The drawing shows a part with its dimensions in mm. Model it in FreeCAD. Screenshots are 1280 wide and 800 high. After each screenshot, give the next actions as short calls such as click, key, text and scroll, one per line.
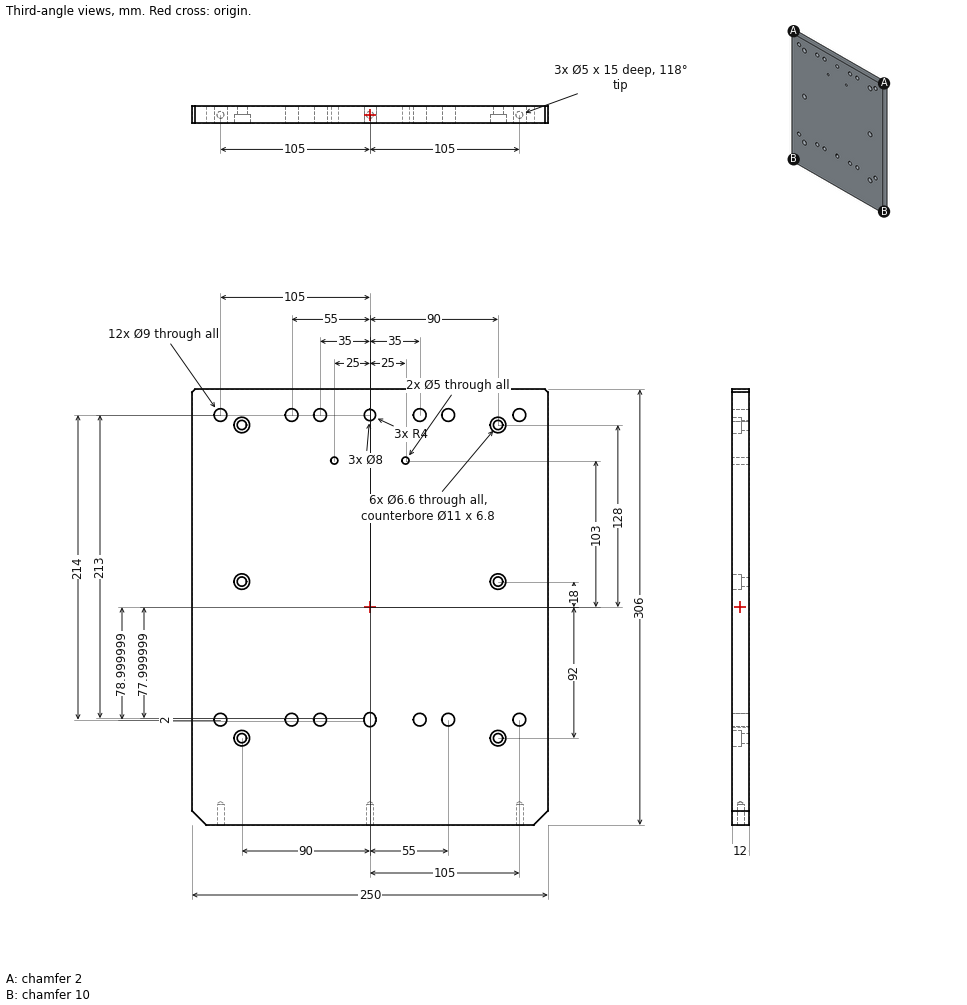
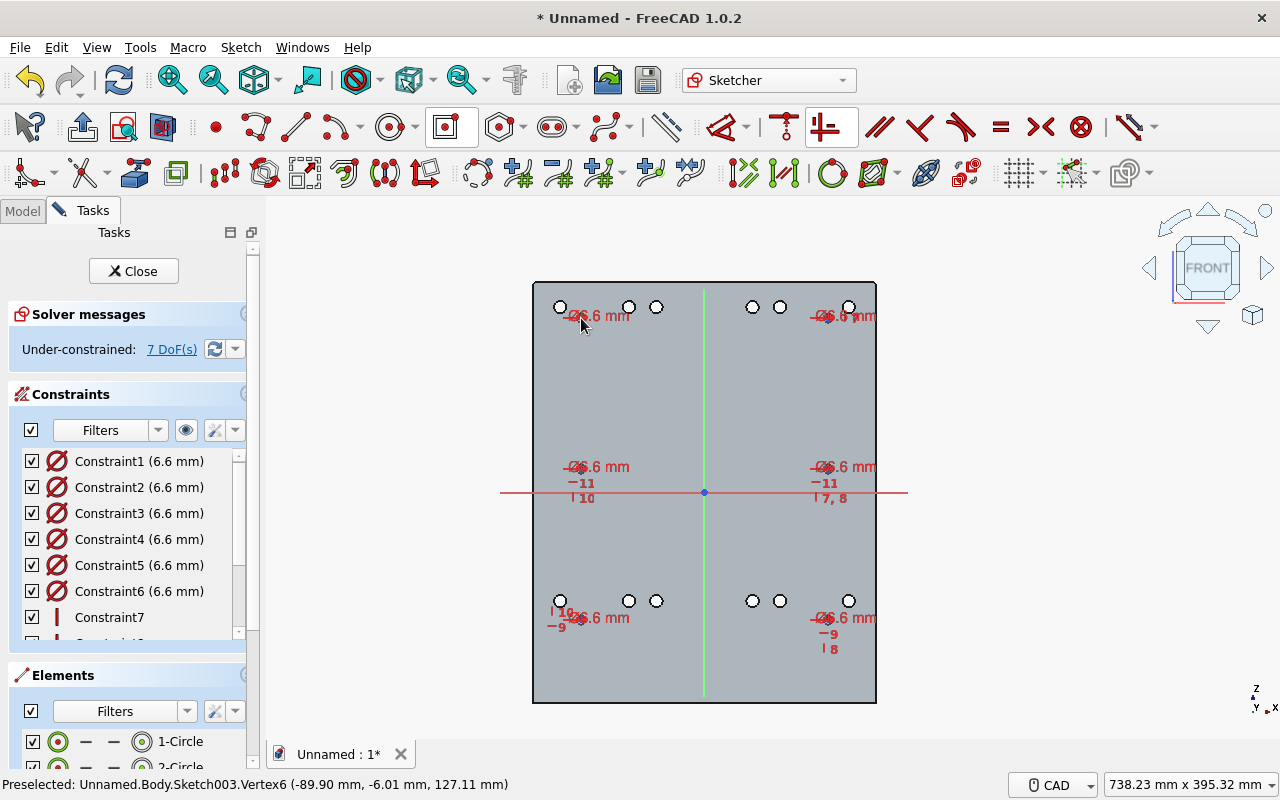
click(852, 128)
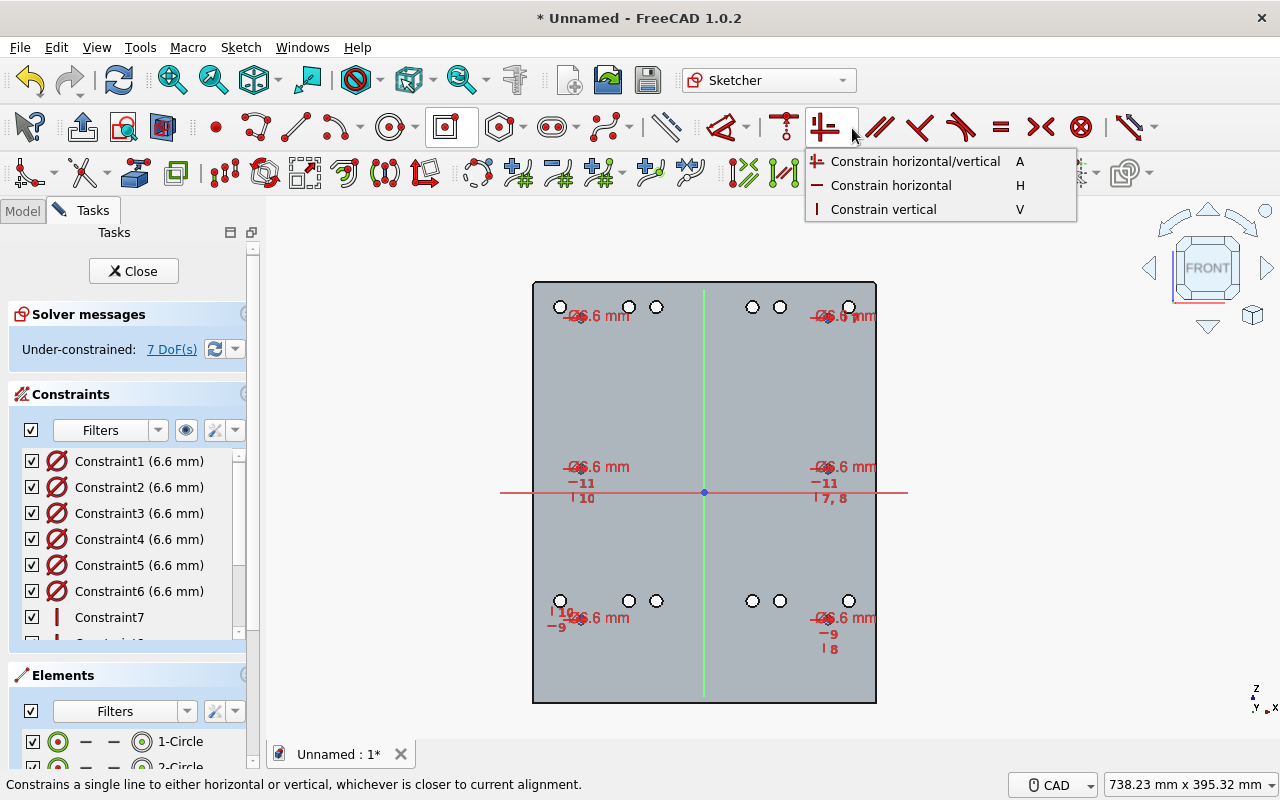
click(941, 209)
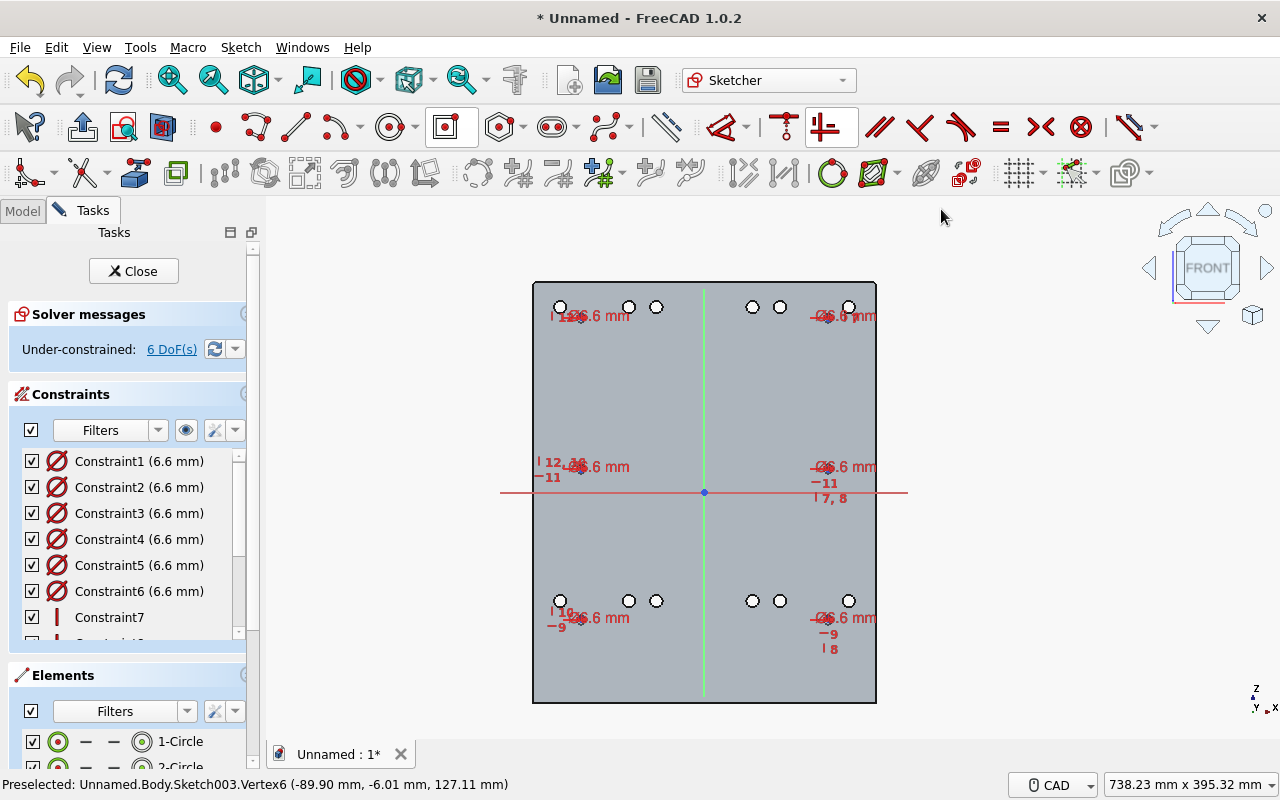
click(828, 318)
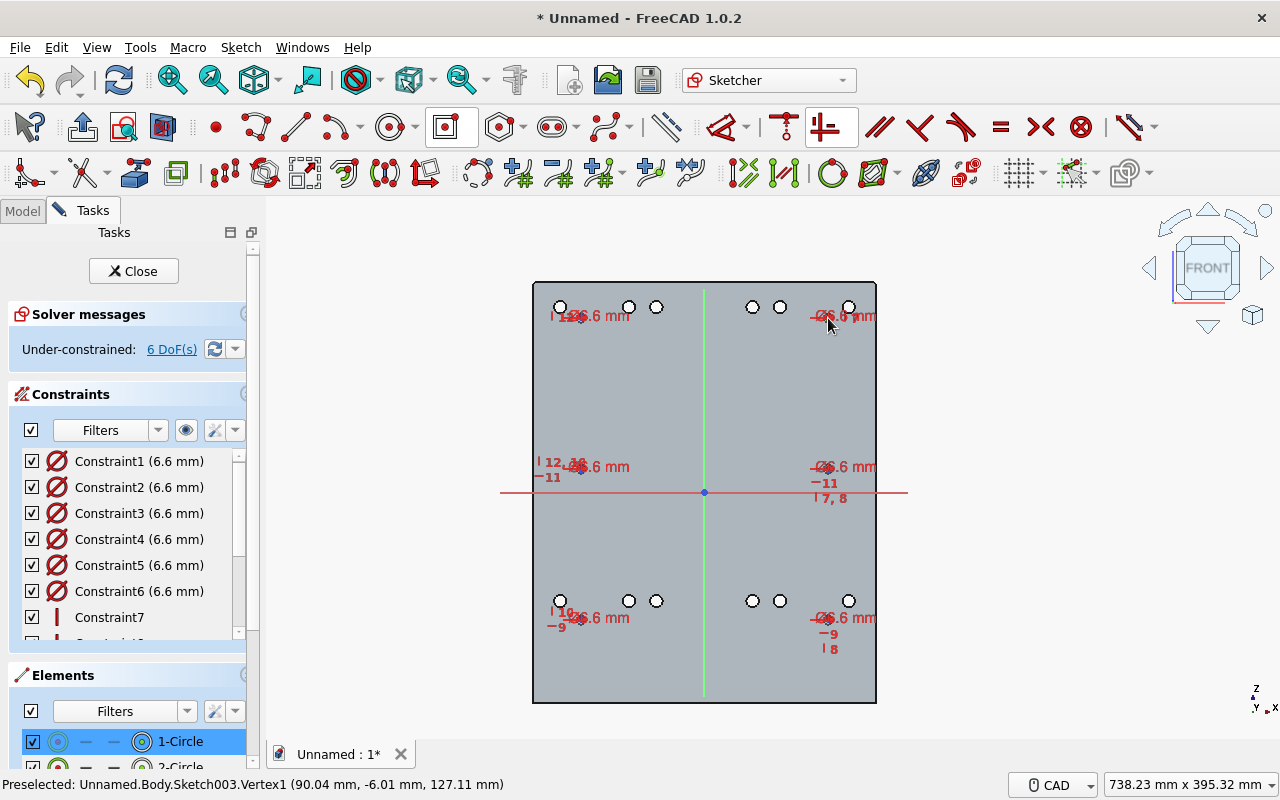
click(581, 318)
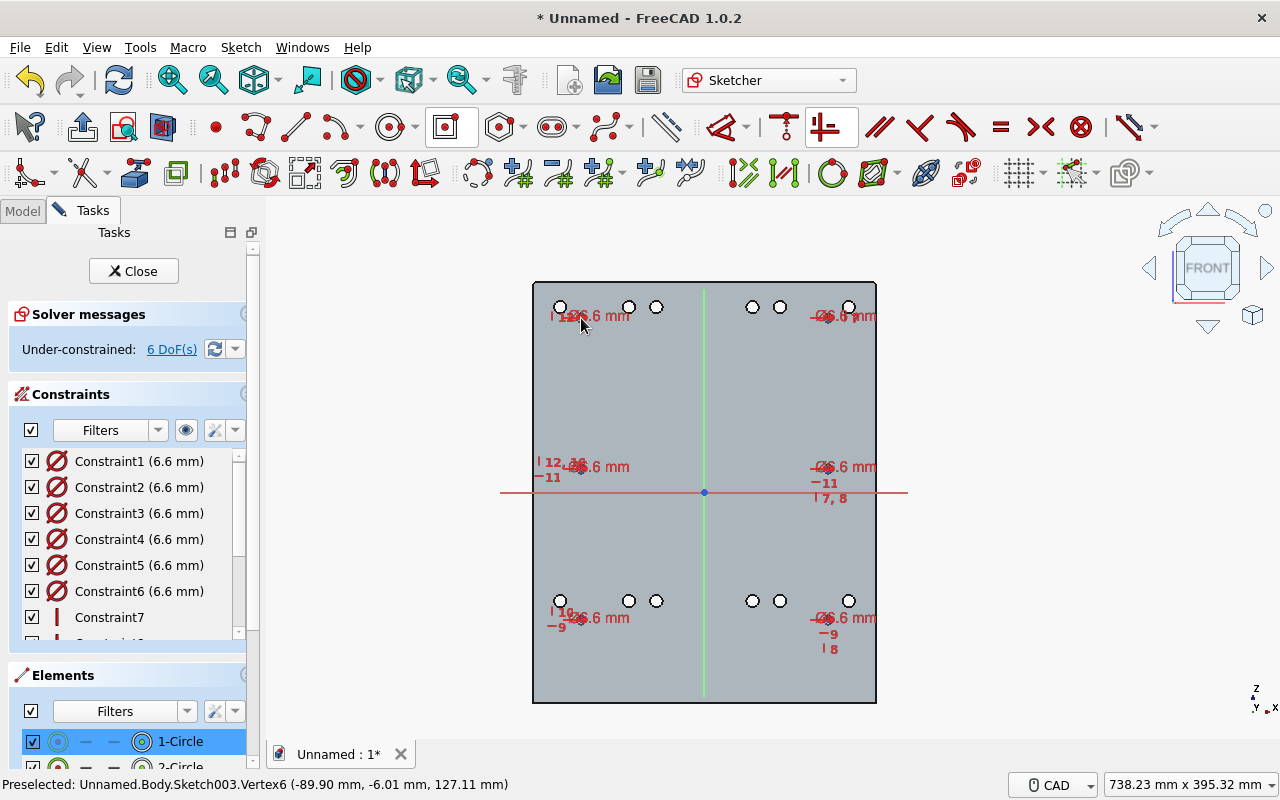
key(h)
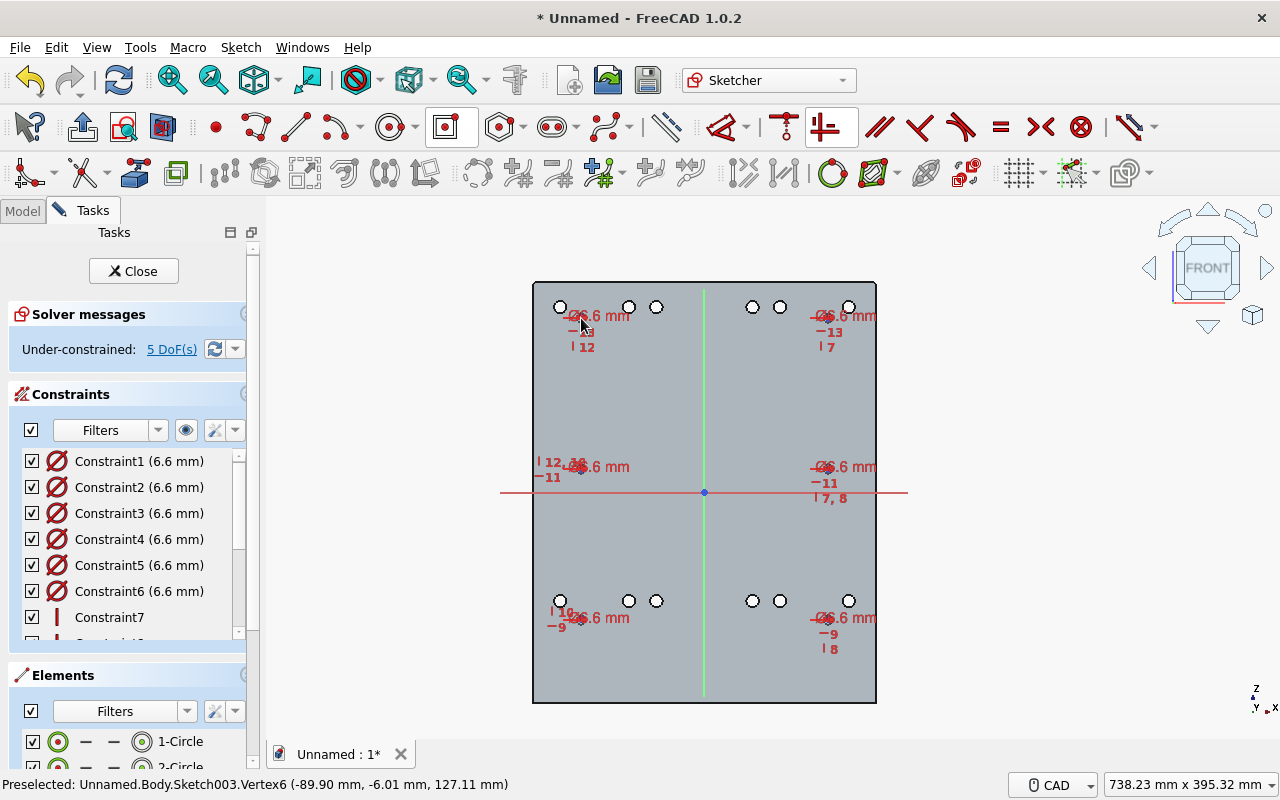
click(722, 128)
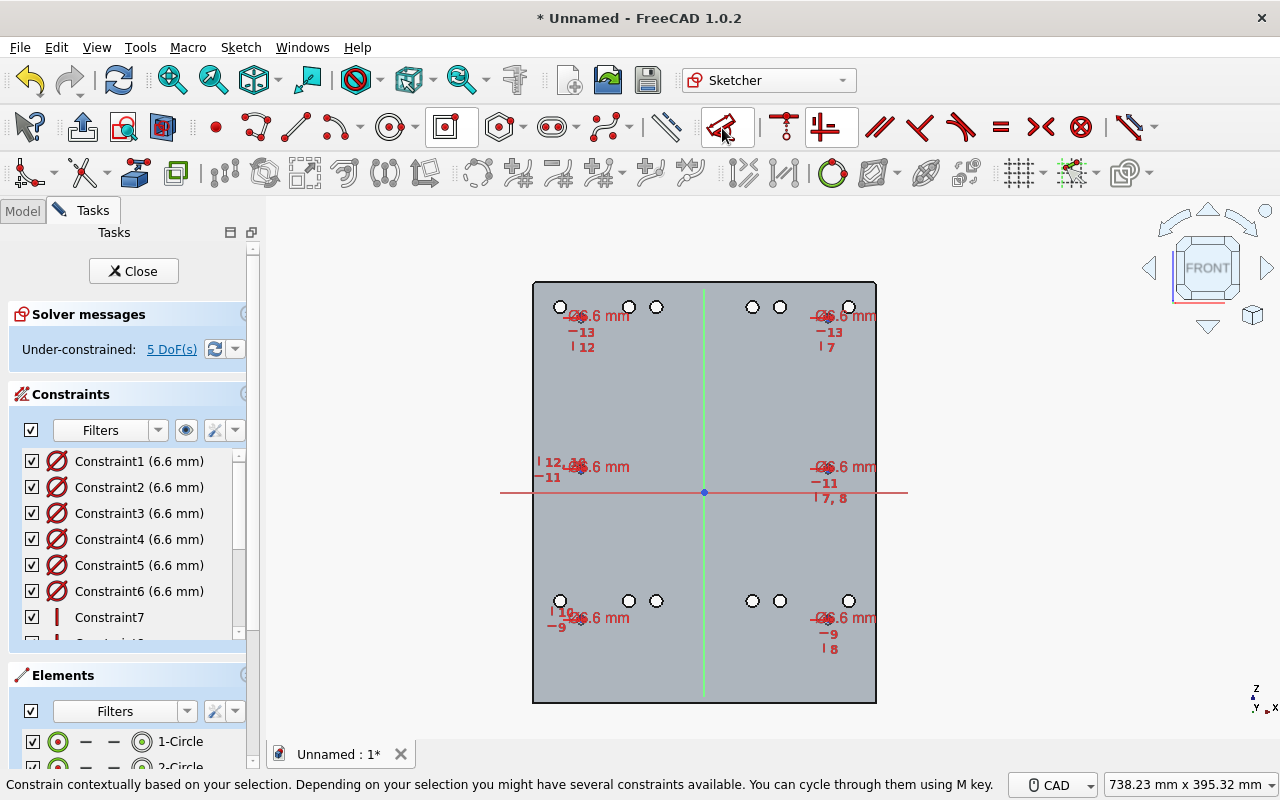
click(828, 318)
click(766, 284)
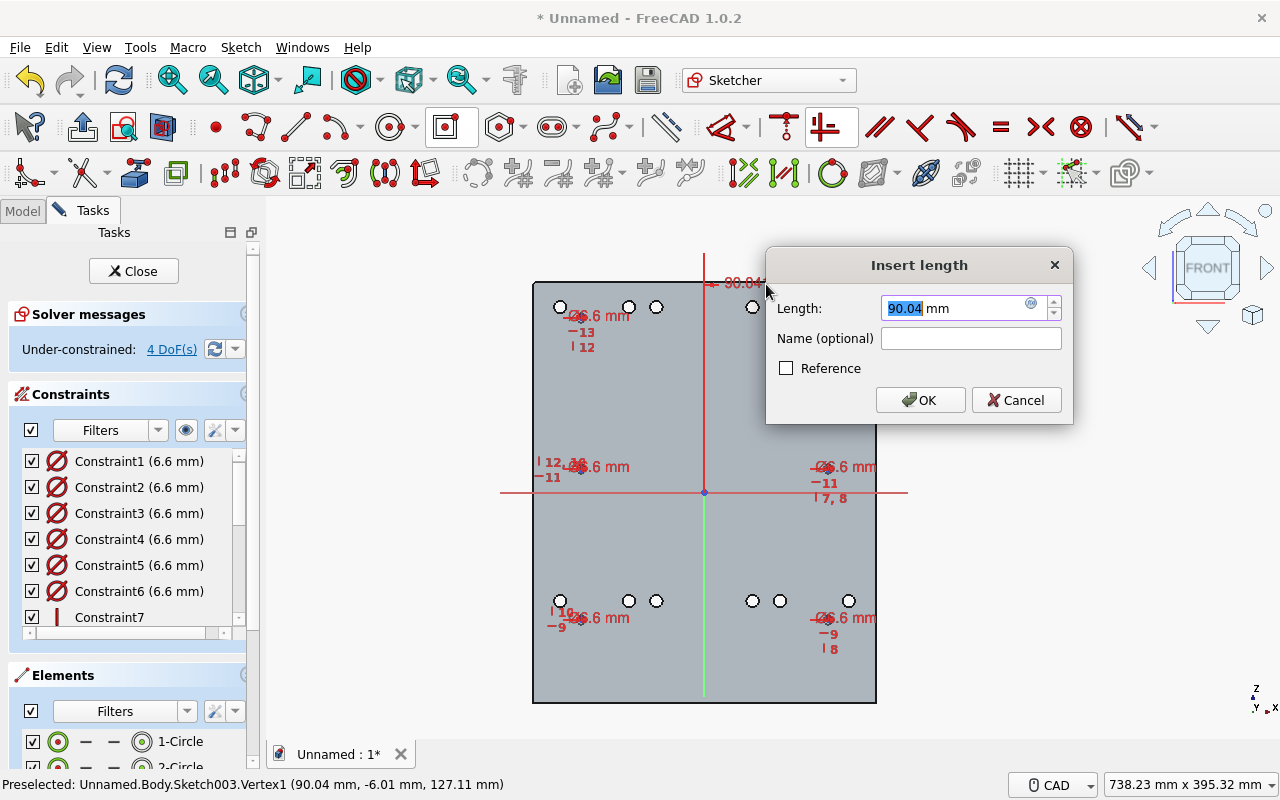
text(90)
key(Return)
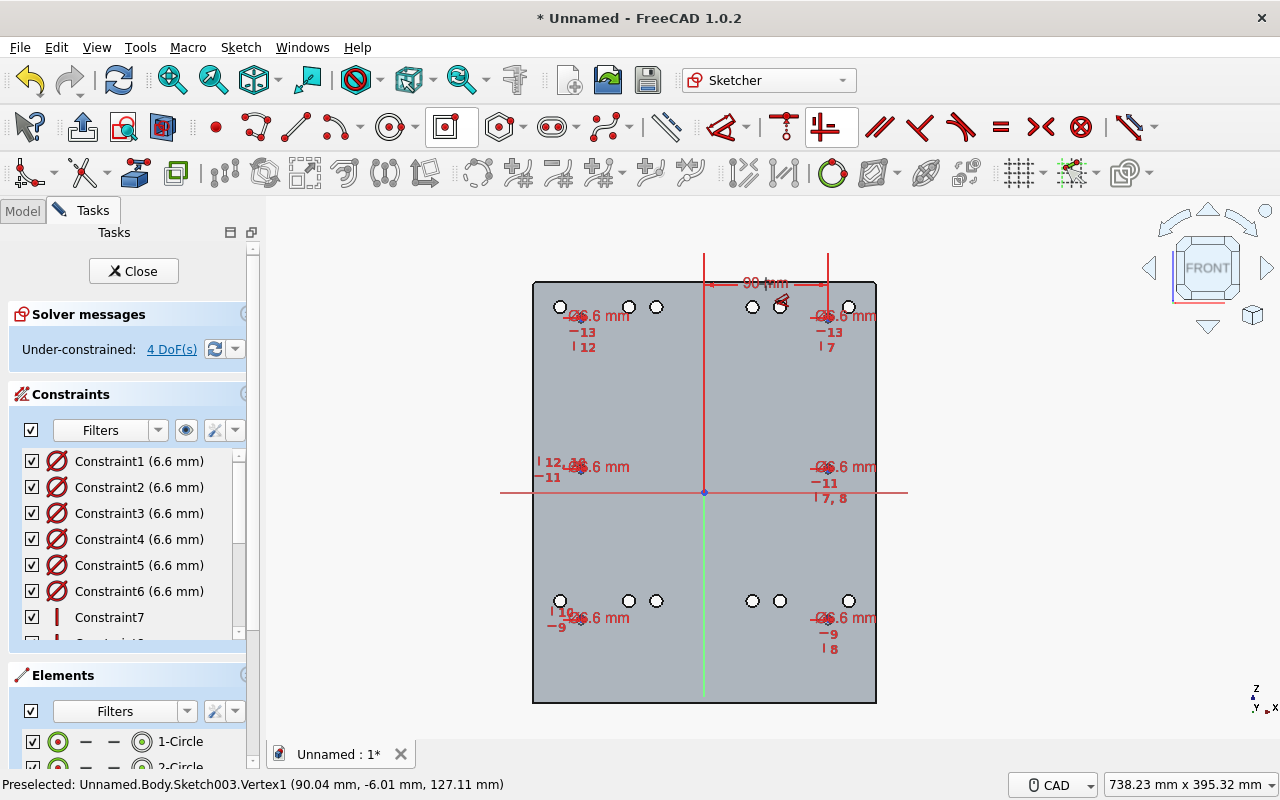
scroll(828, 469, up, 3)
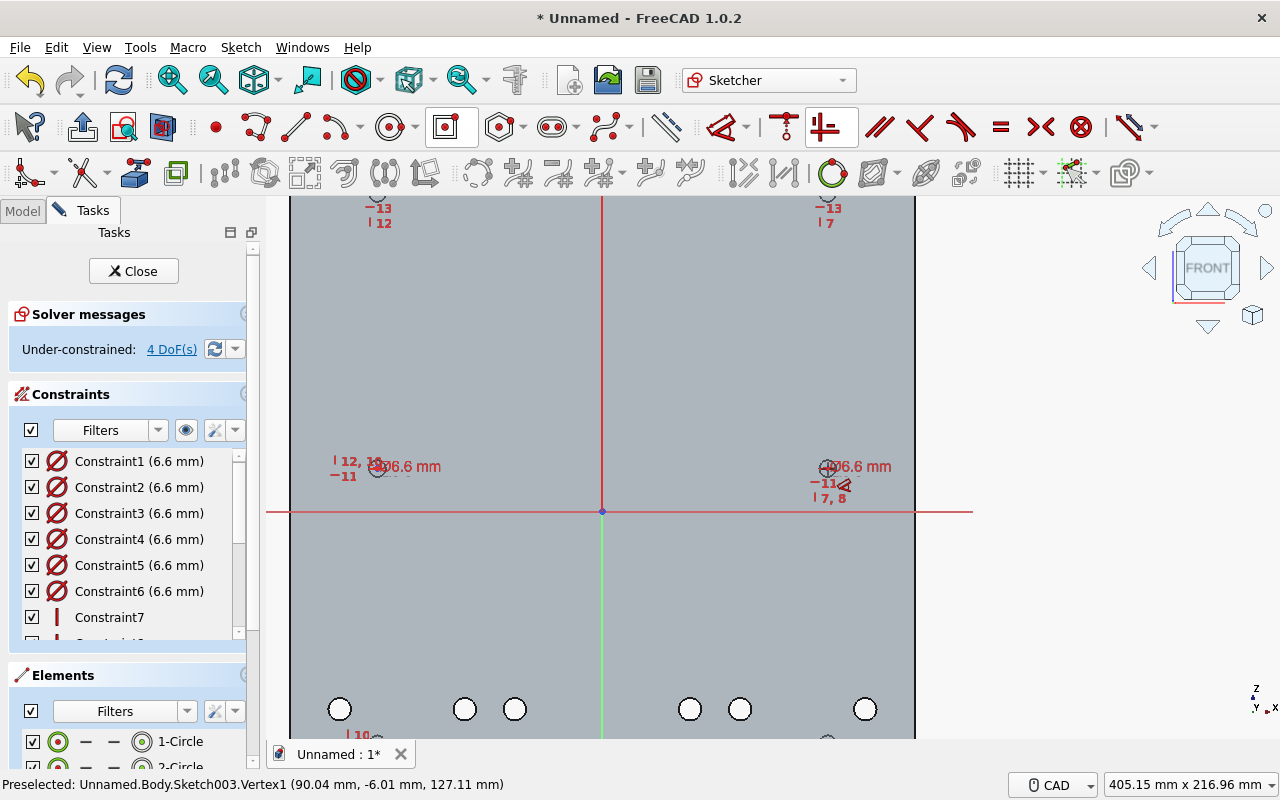
click(828, 469)
click(862, 490)